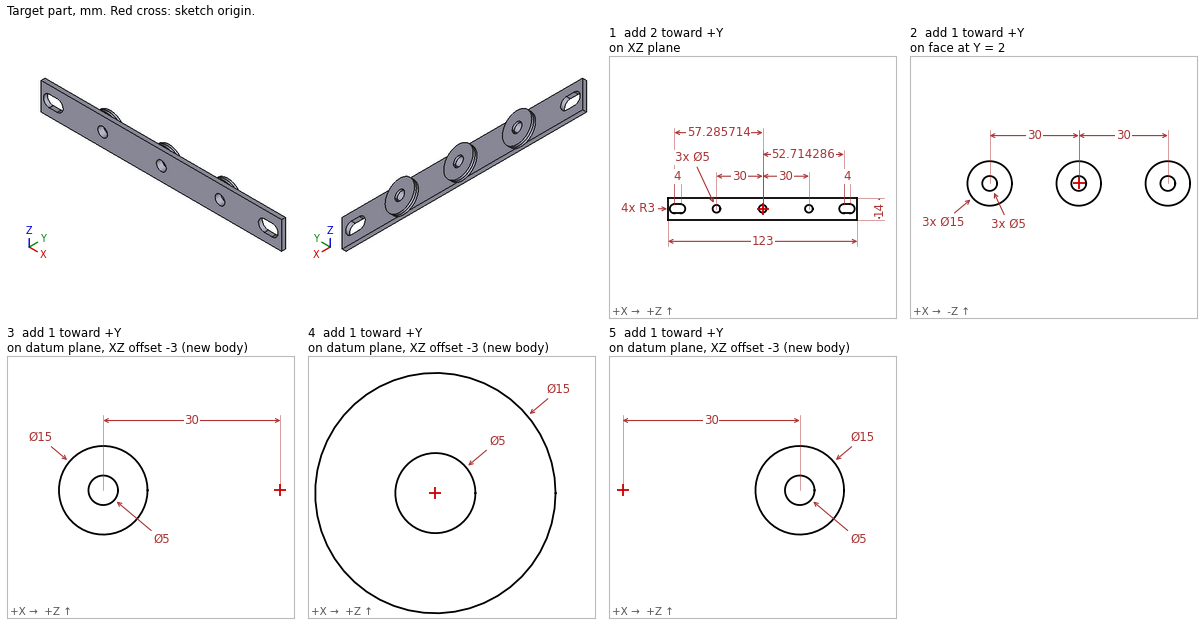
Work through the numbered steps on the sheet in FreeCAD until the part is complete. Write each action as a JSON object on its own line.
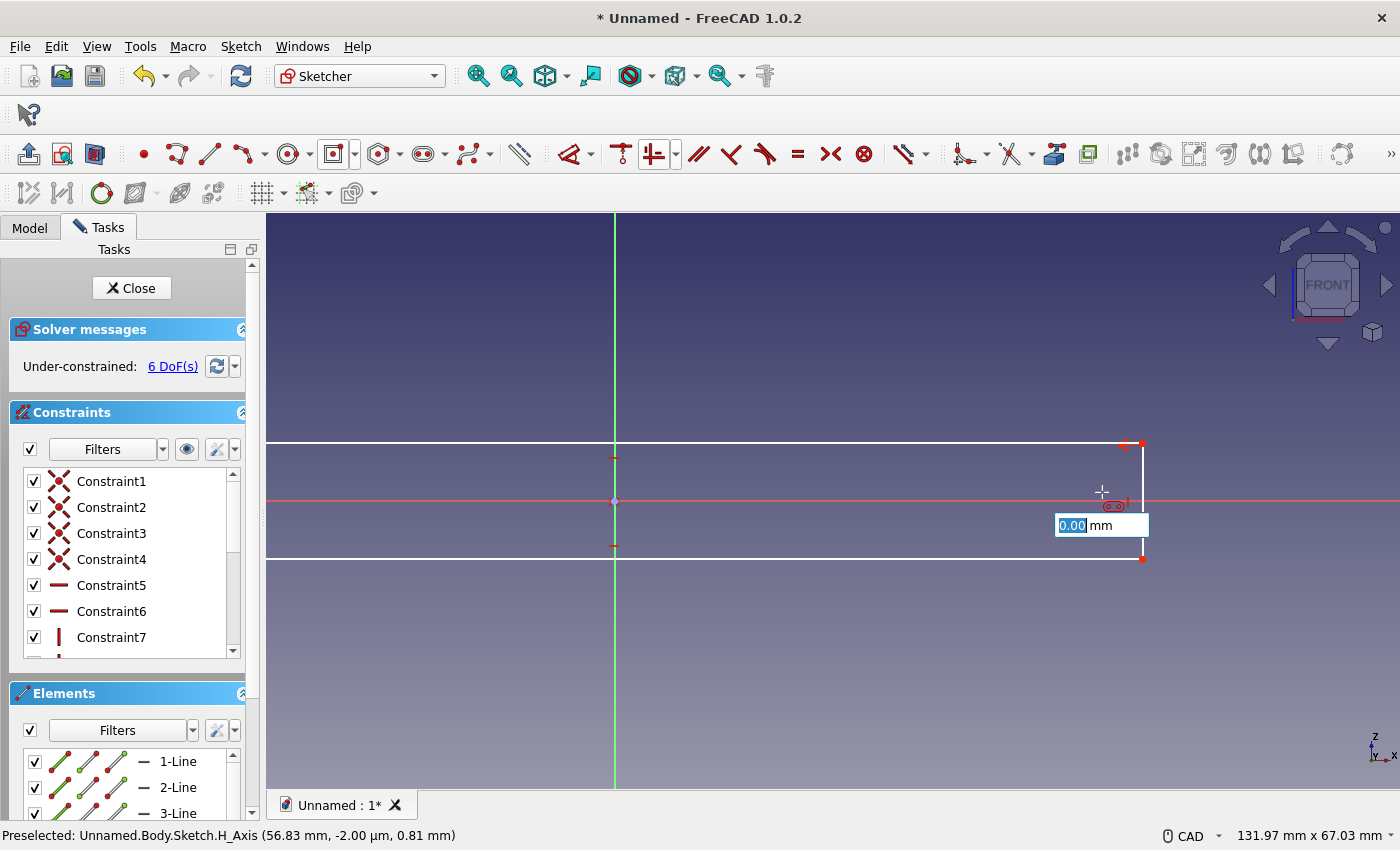
{"action": "left_click", "coordinate": [1085, 527]}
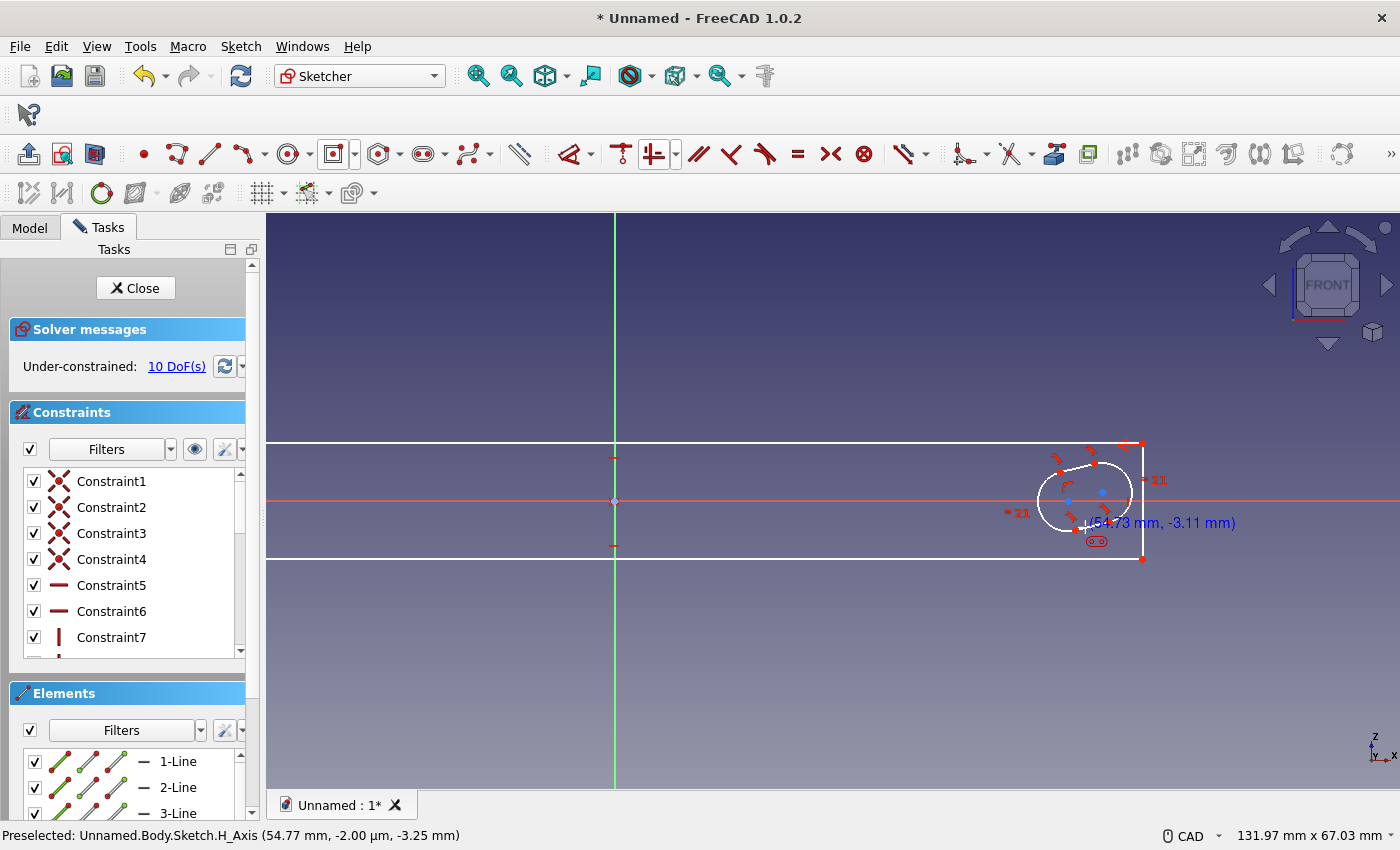
{"action": "left_click", "coordinate": [288, 154]}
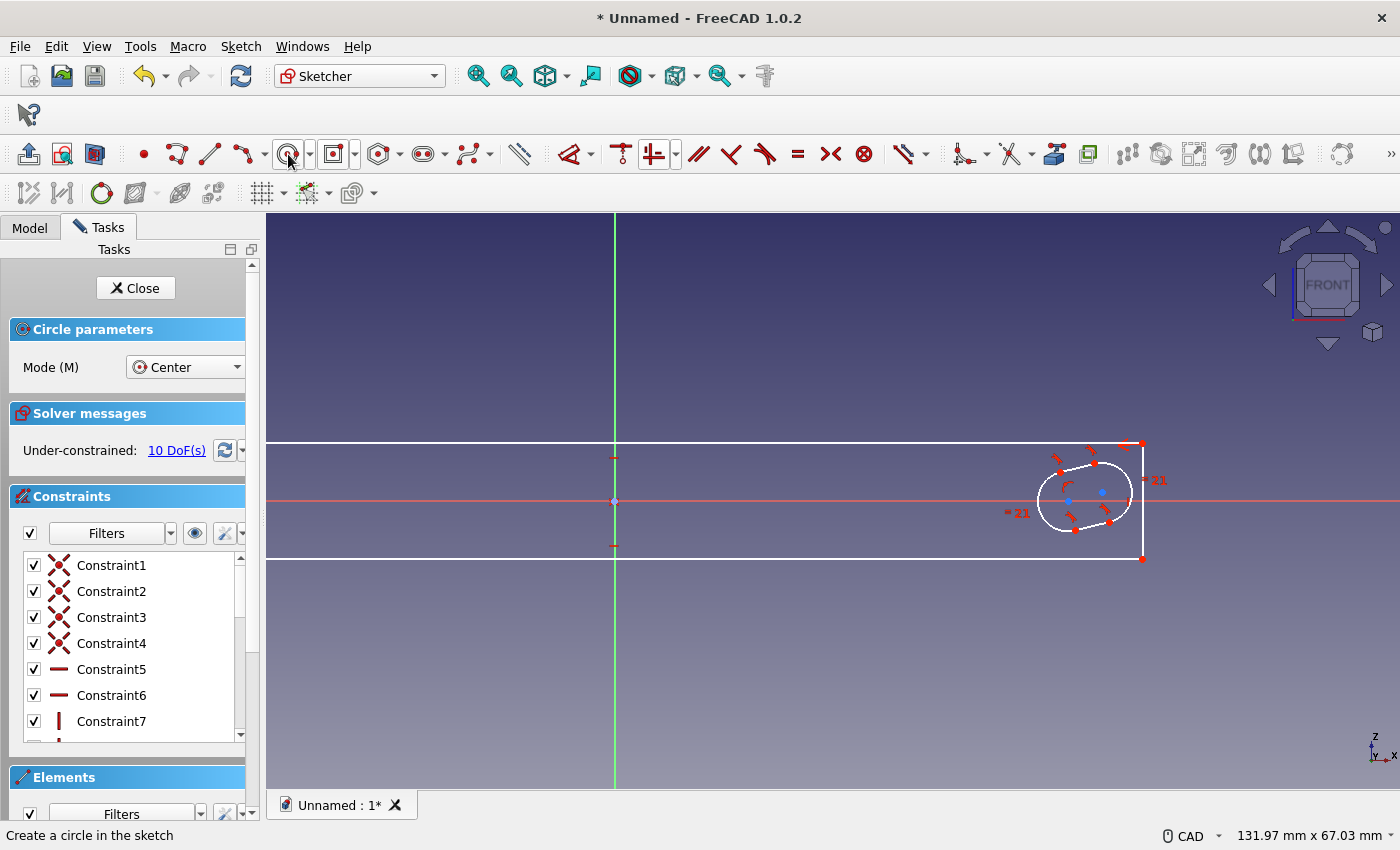
{"action": "left_click", "coordinate": [357, 501]}
{"action": "left_click", "coordinate": [372, 486]}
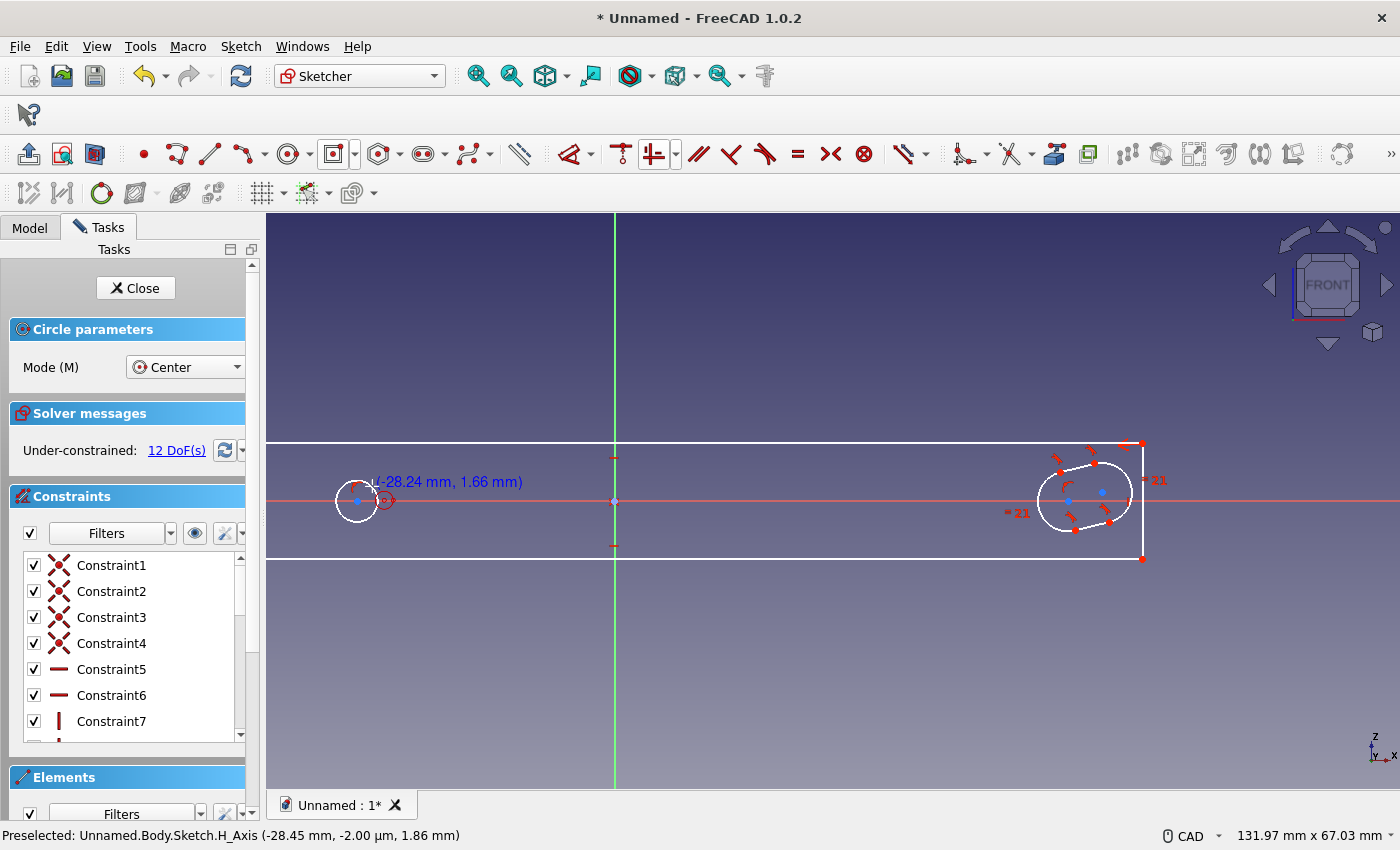
{"action": "left_click", "coordinate": [615, 501]}
{"action": "left_click", "coordinate": [630, 486]}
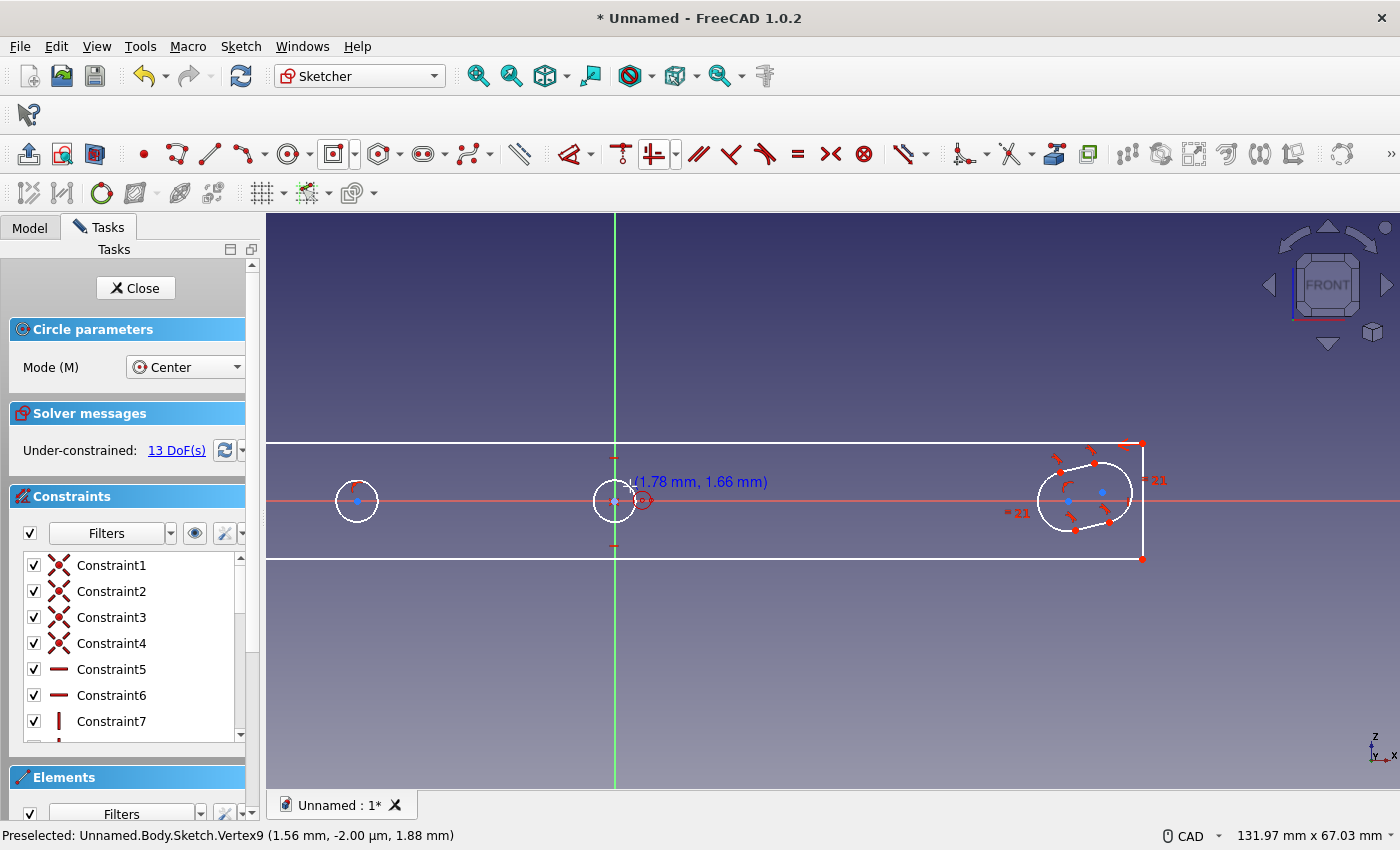
{"action": "left_click", "coordinate": [872, 501]}
{"action": "left_click", "coordinate": [888, 486]}
{"action": "key", "text": "Escape"}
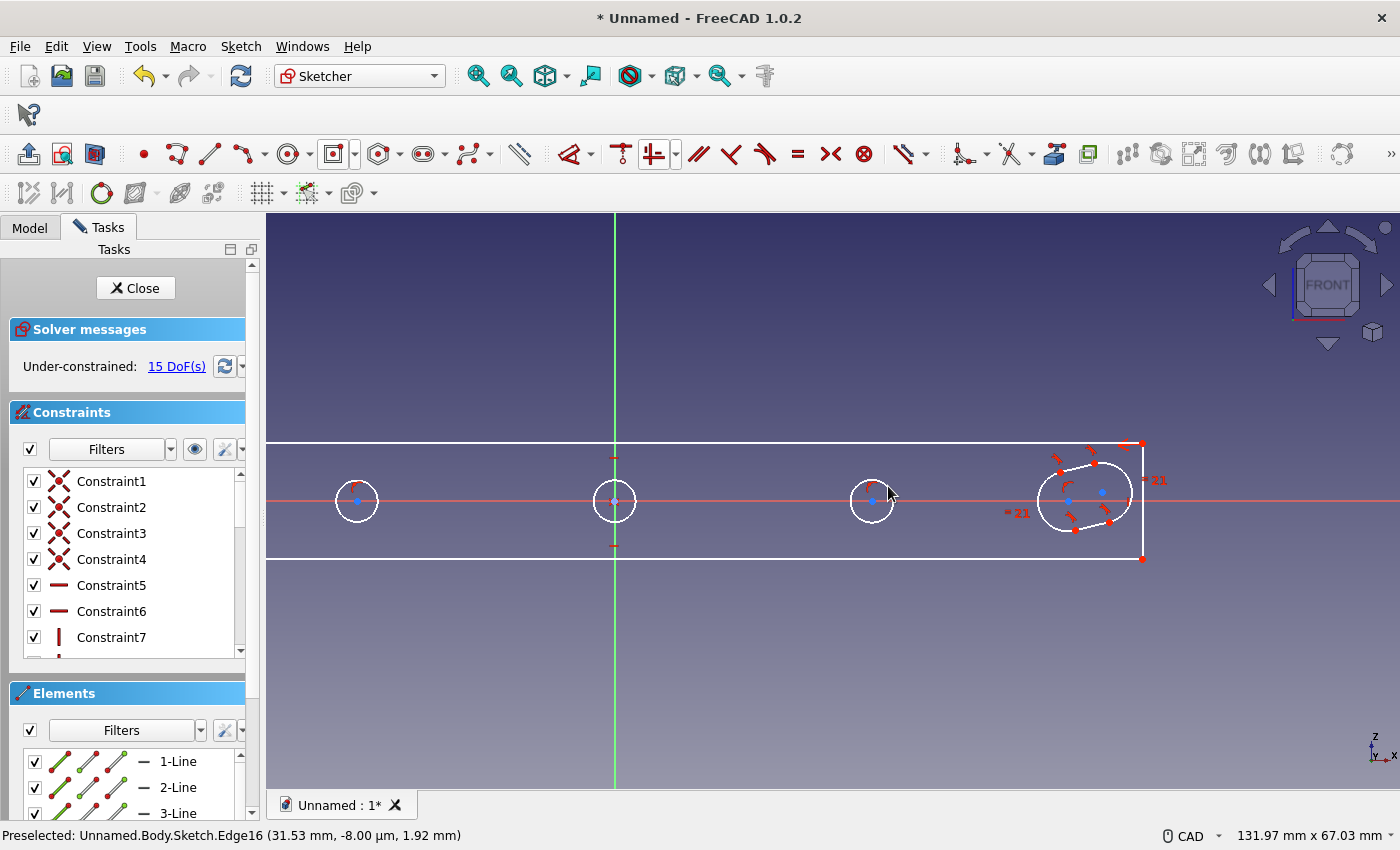
{"action": "scroll", "coordinate": [1069, 500], "scroll_direction": "down", "scroll_amount": 2}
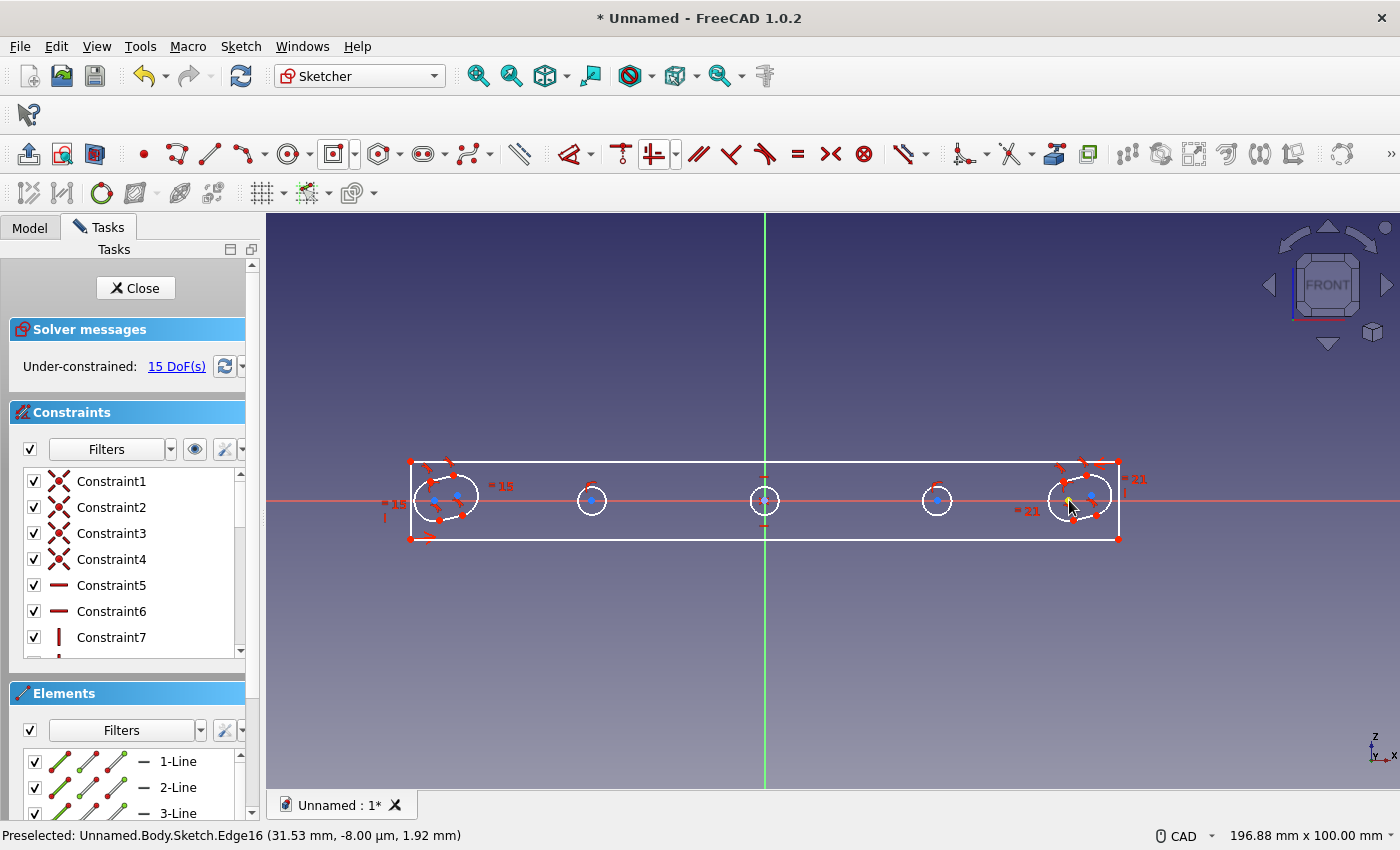
{"action": "scroll", "coordinate": [437, 480], "scroll_direction": "up", "scroll_amount": 4}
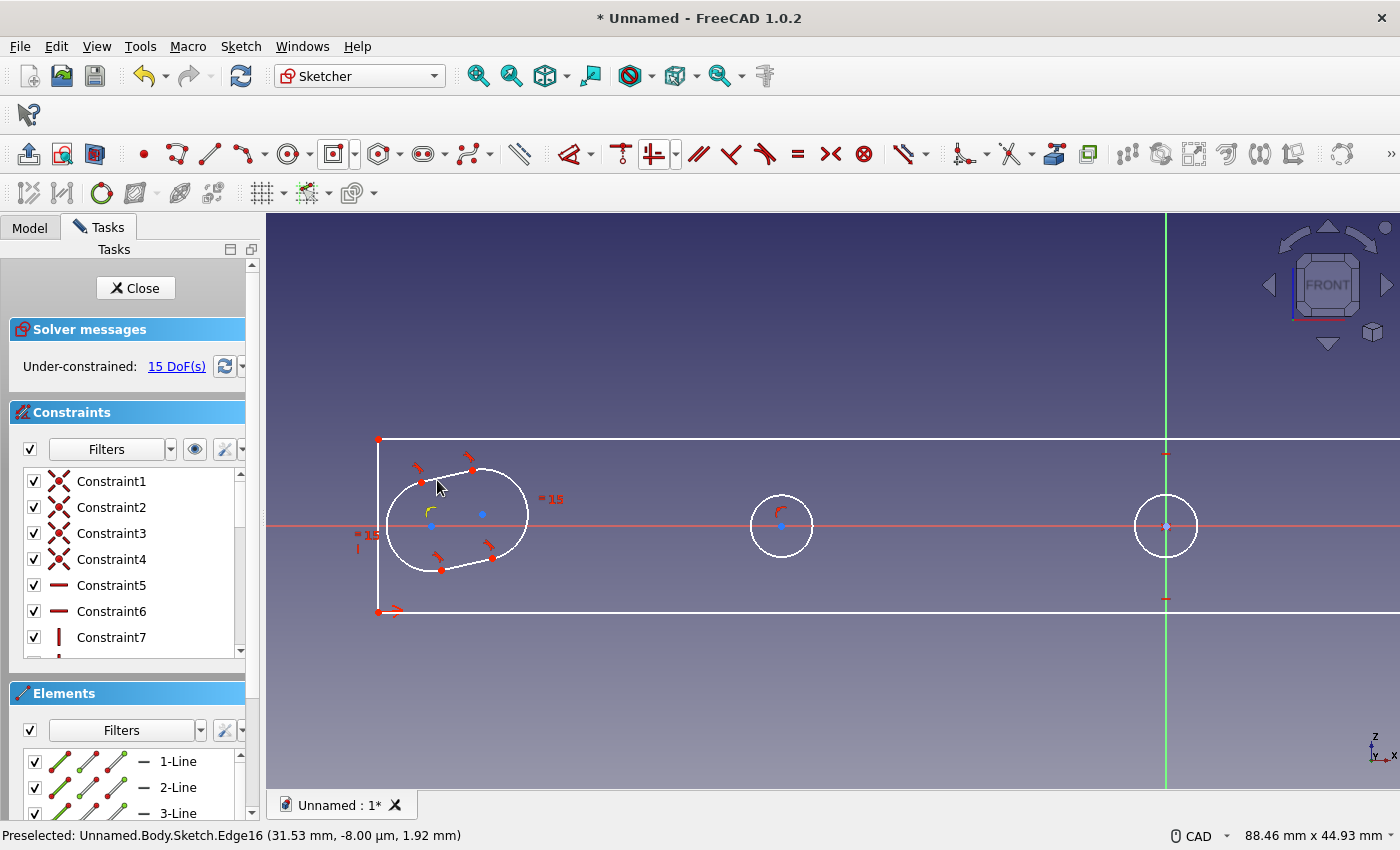
{"action": "left_click", "coordinate": [437, 479]}